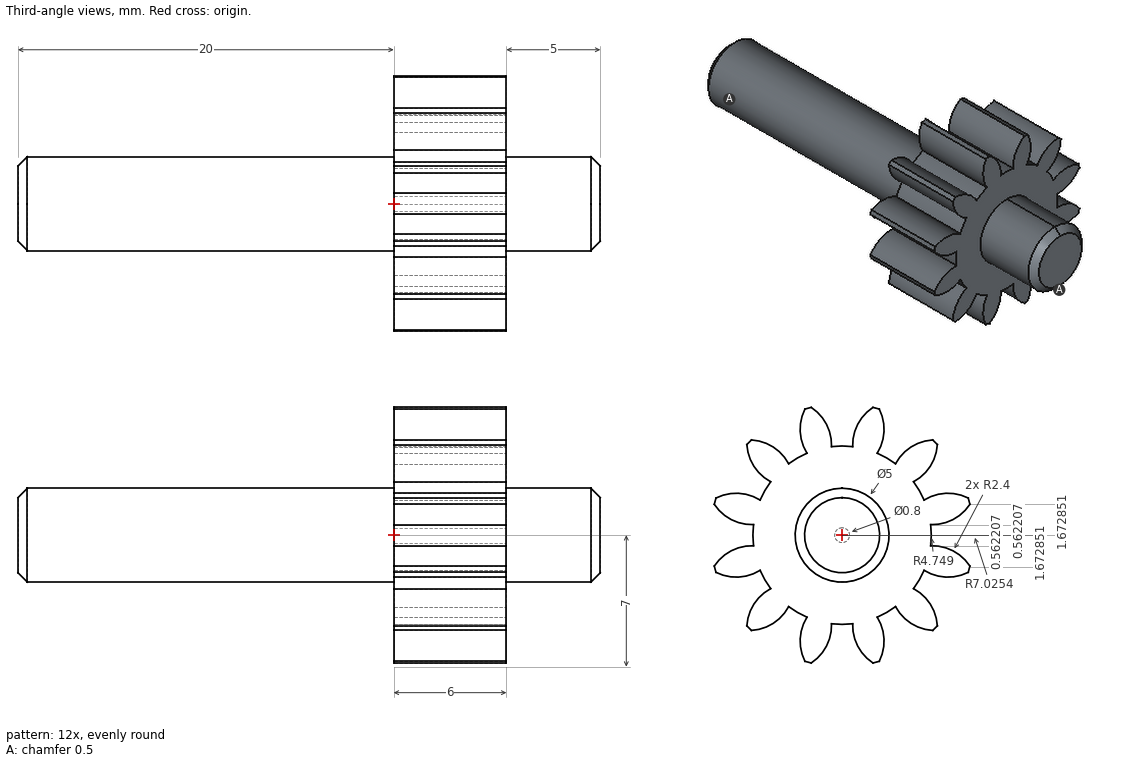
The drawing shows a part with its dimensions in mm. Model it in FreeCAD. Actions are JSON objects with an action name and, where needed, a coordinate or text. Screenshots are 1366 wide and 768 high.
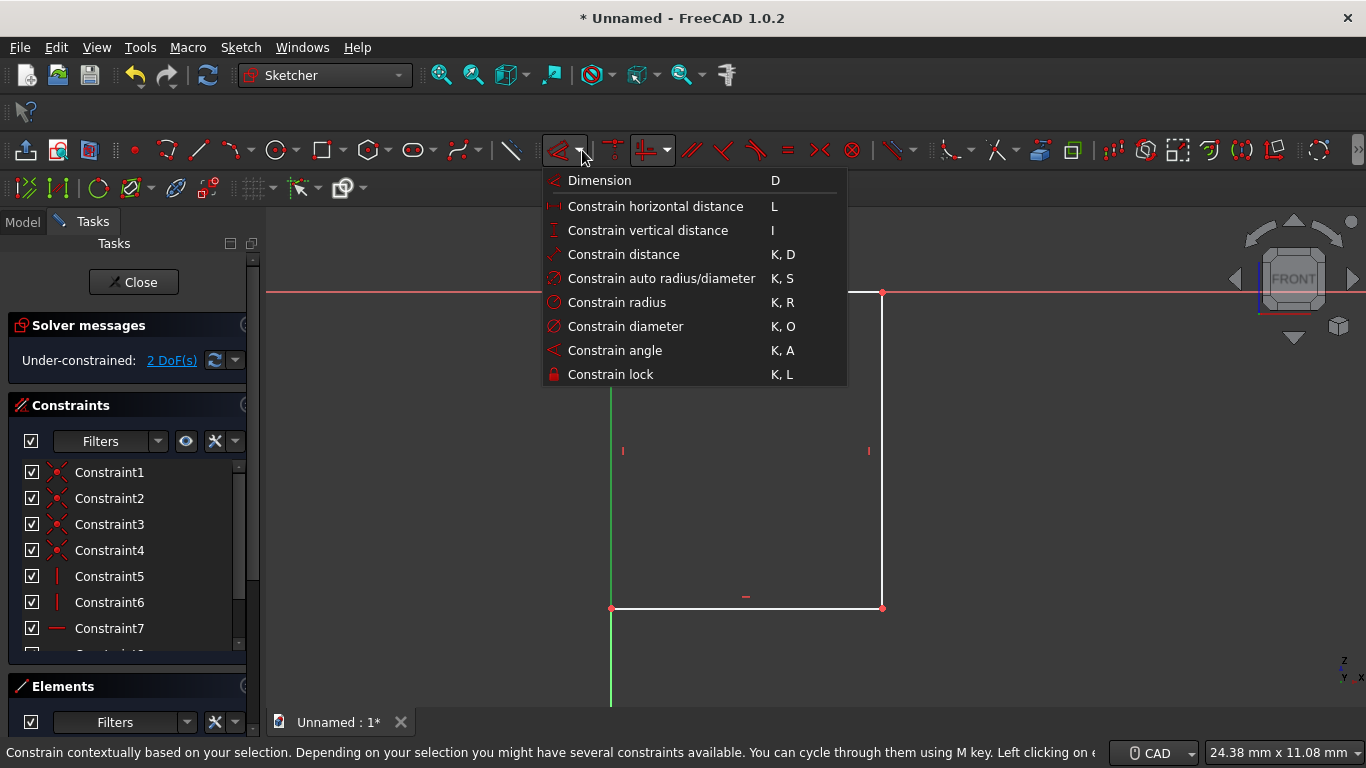
{"action": "left_click", "coordinate": [695, 230]}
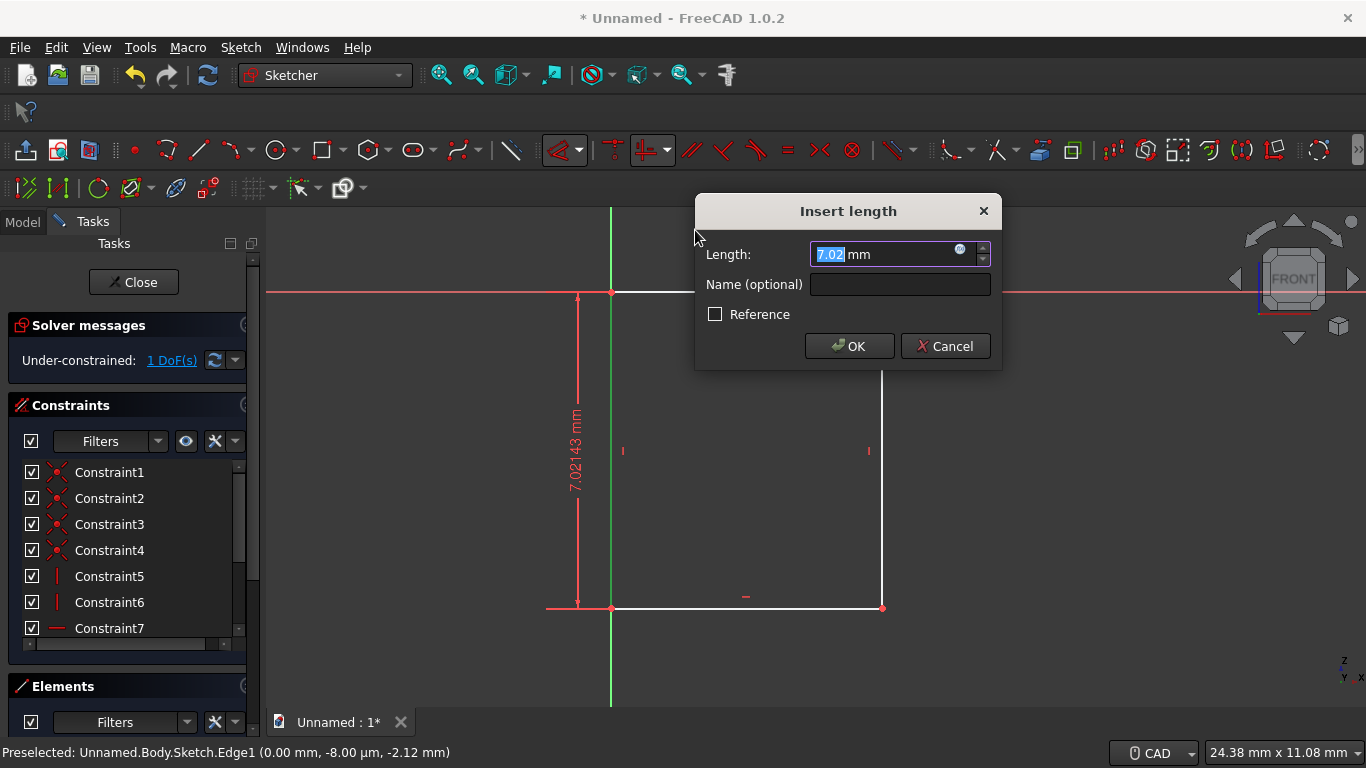
{"action": "type", "text": "7"}
{"action": "key", "text": "Return"}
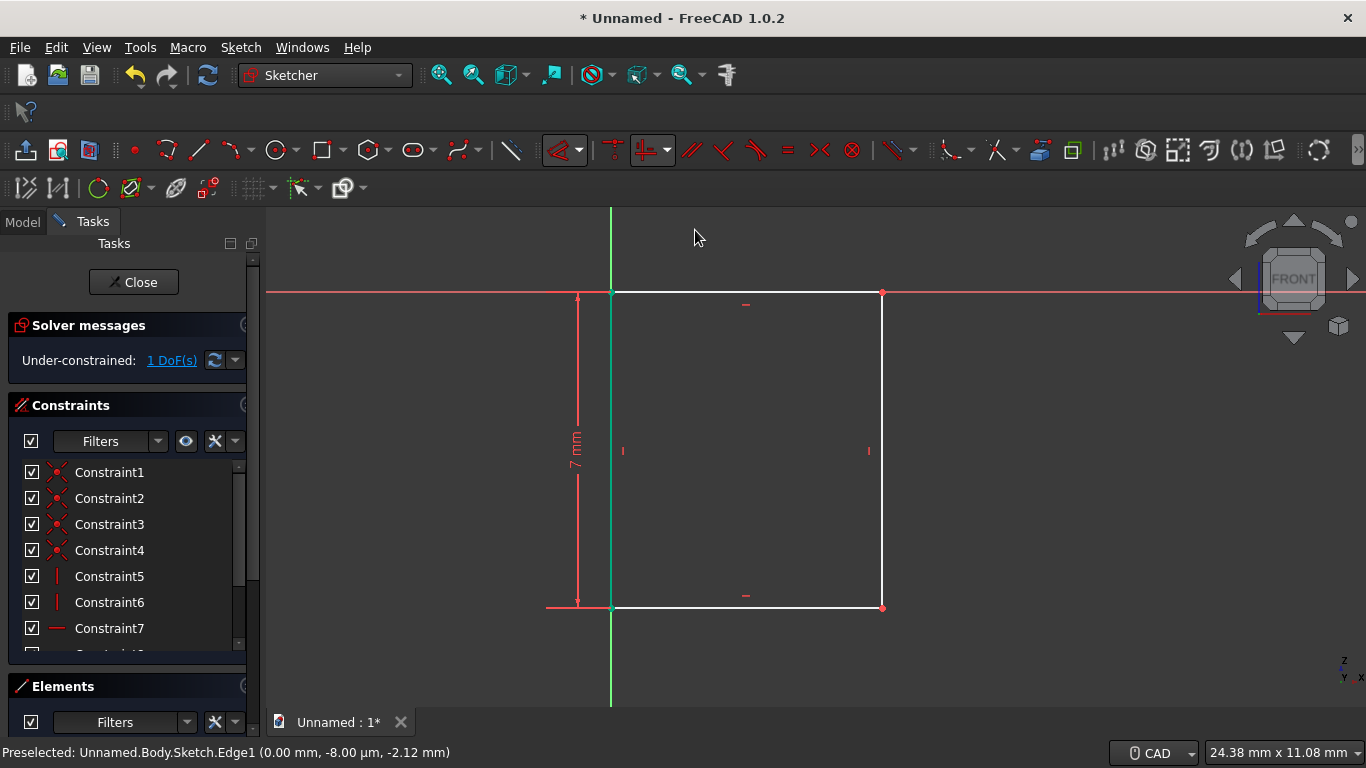
{"action": "left_click", "coordinate": [692, 608]}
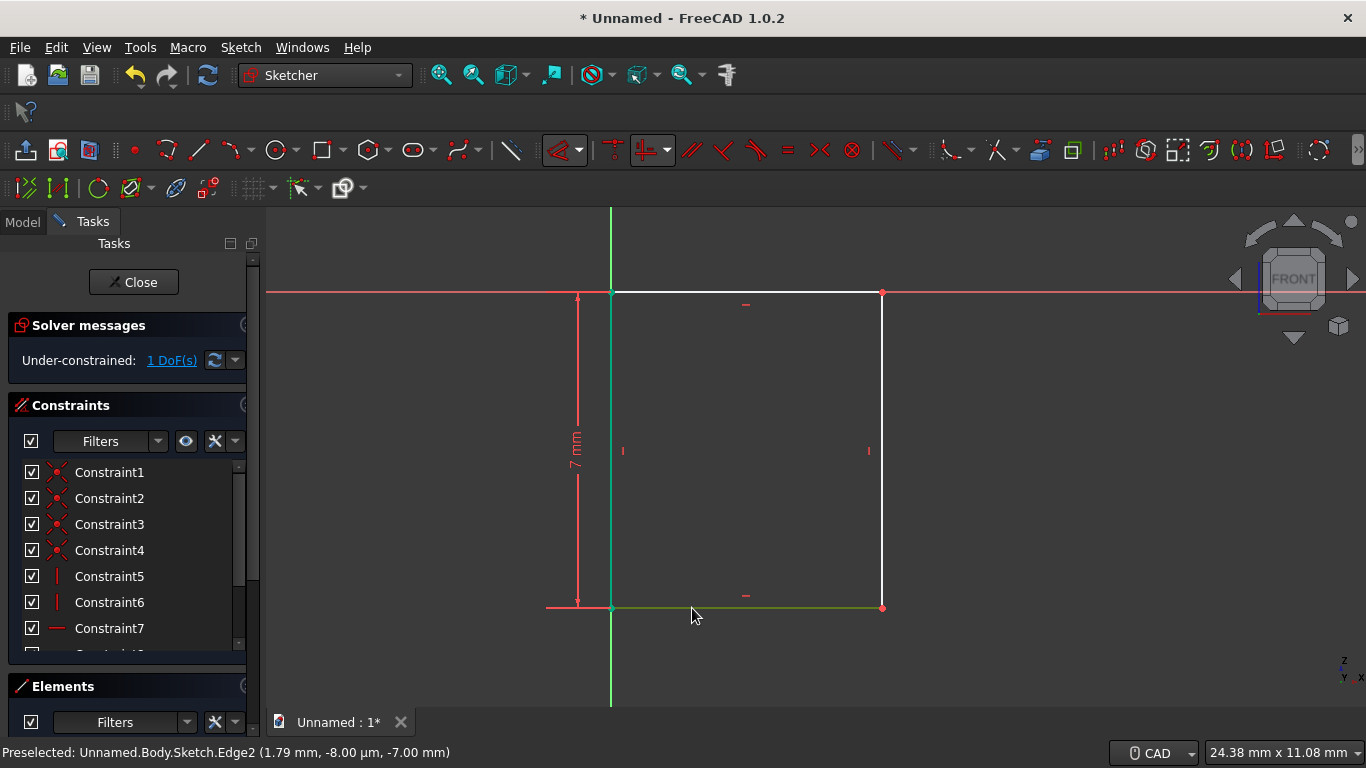
{"action": "key", "text": "l"}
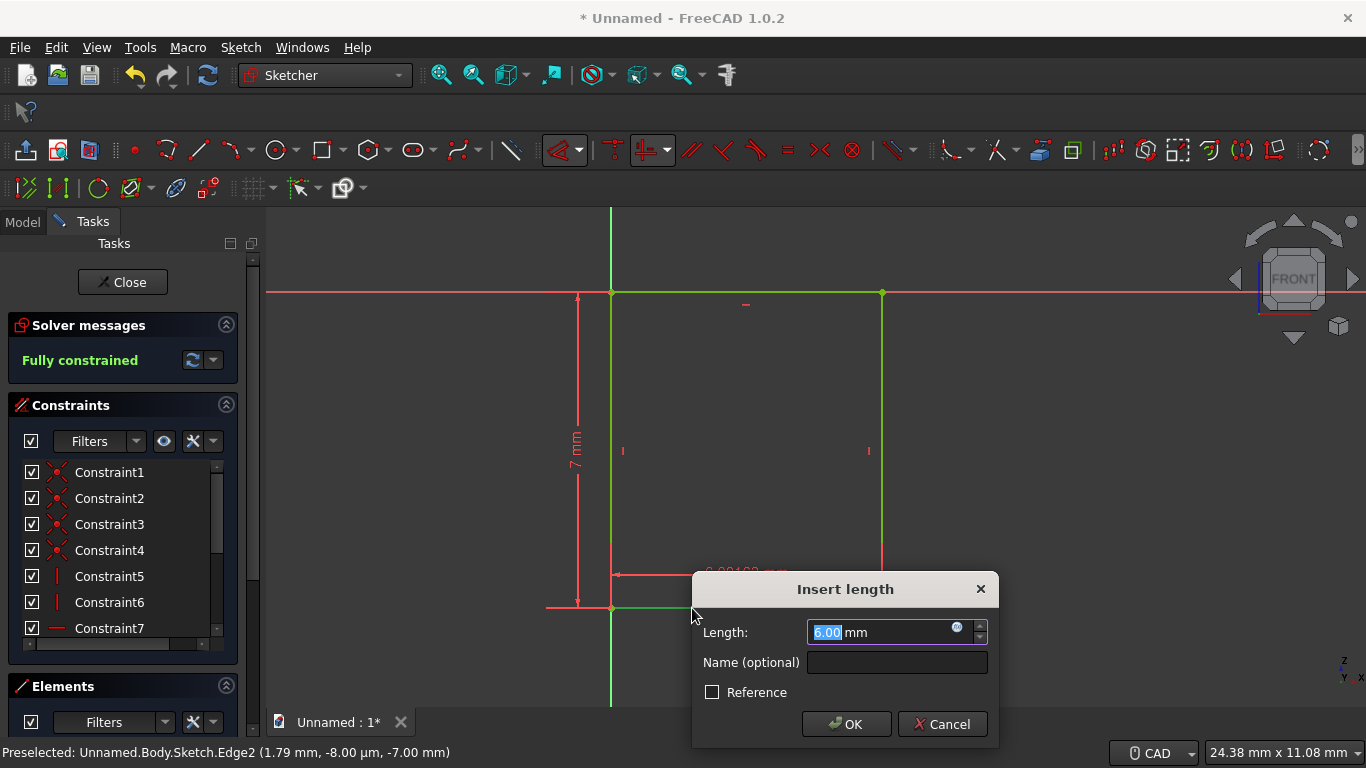
{"action": "type", "text": "6"}
{"action": "key", "text": "Return"}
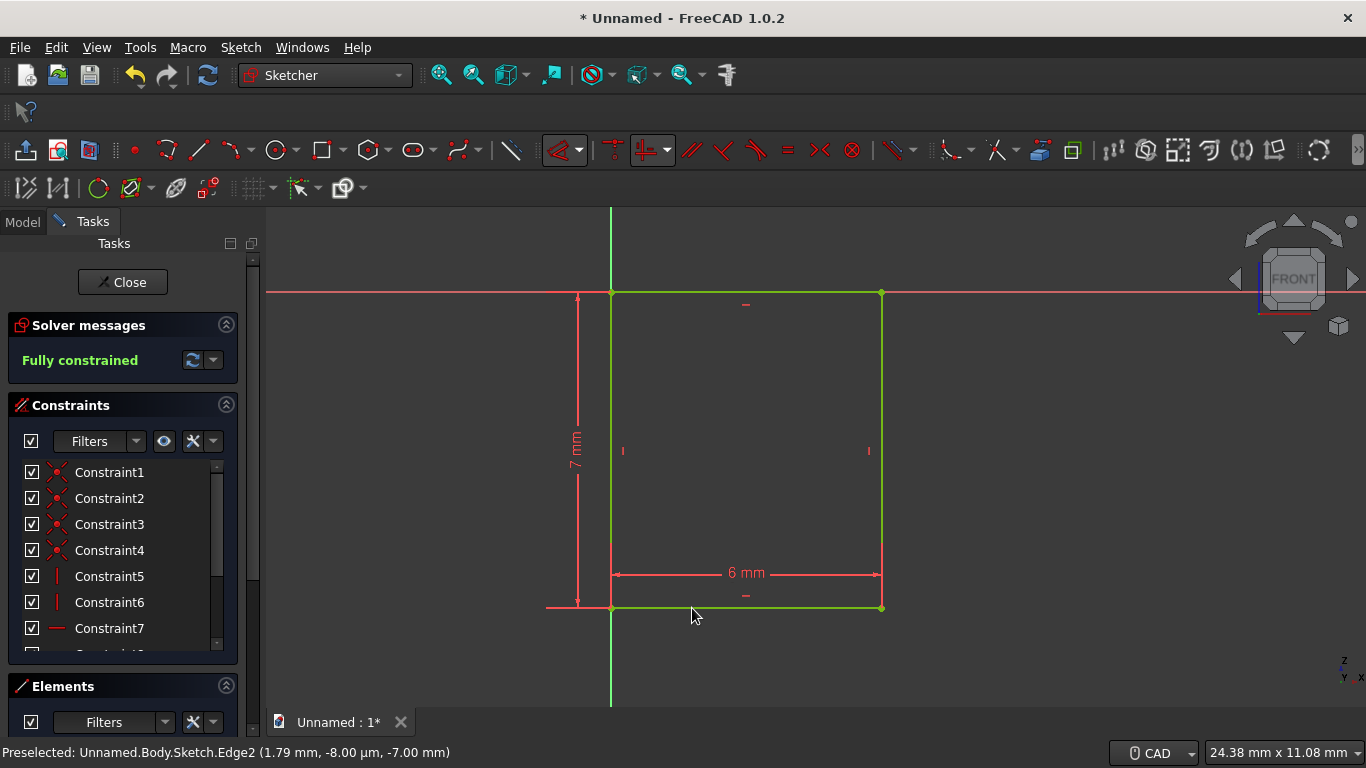
{"action": "left_click", "coordinate": [123, 282]}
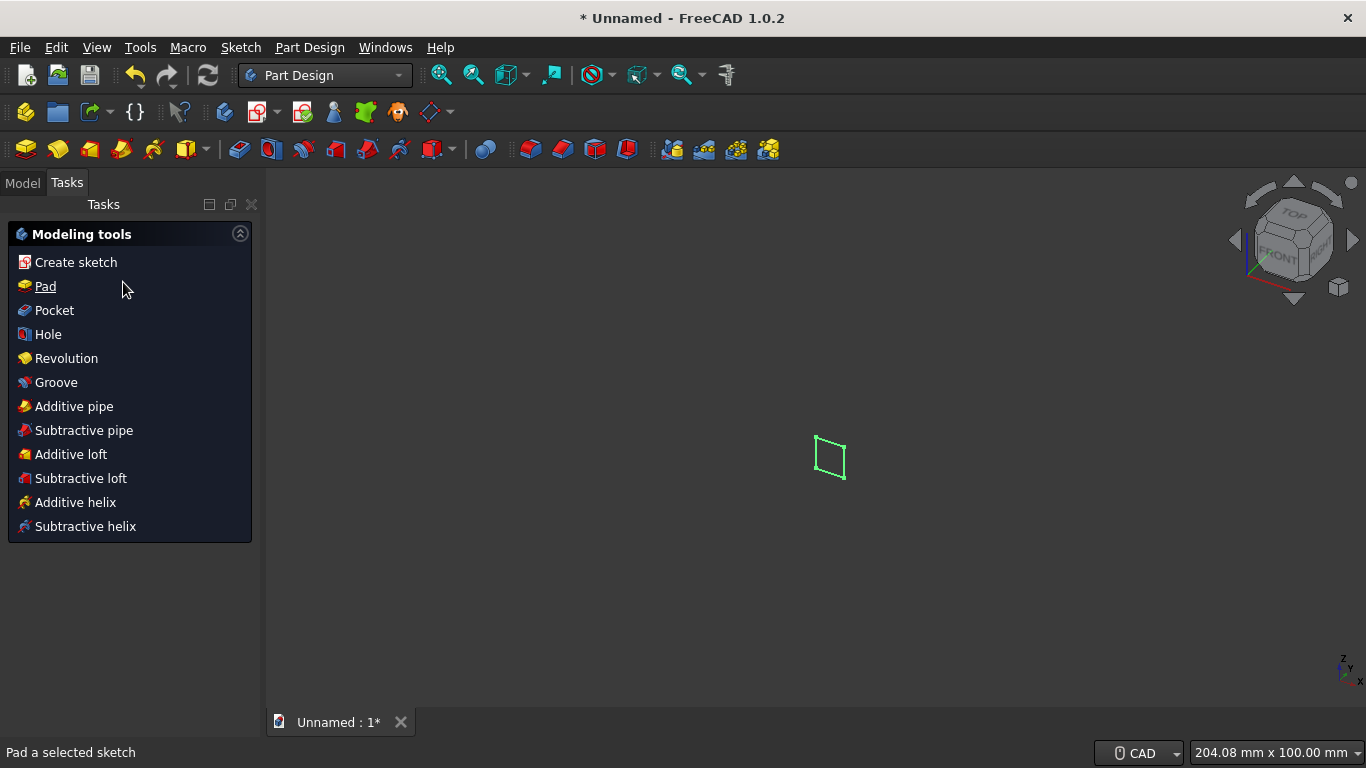
{"action": "left_click", "coordinate": [58, 150]}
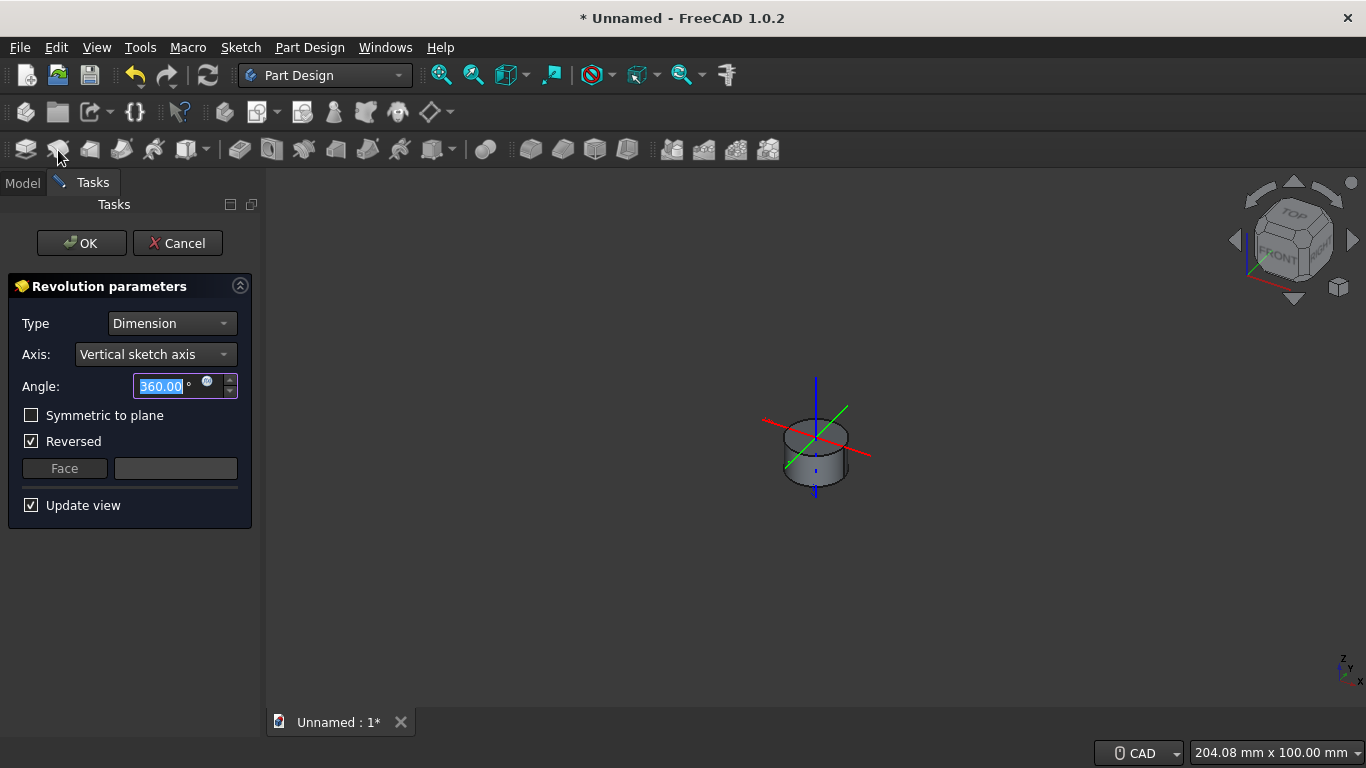
{"action": "left_click", "coordinate": [156, 354]}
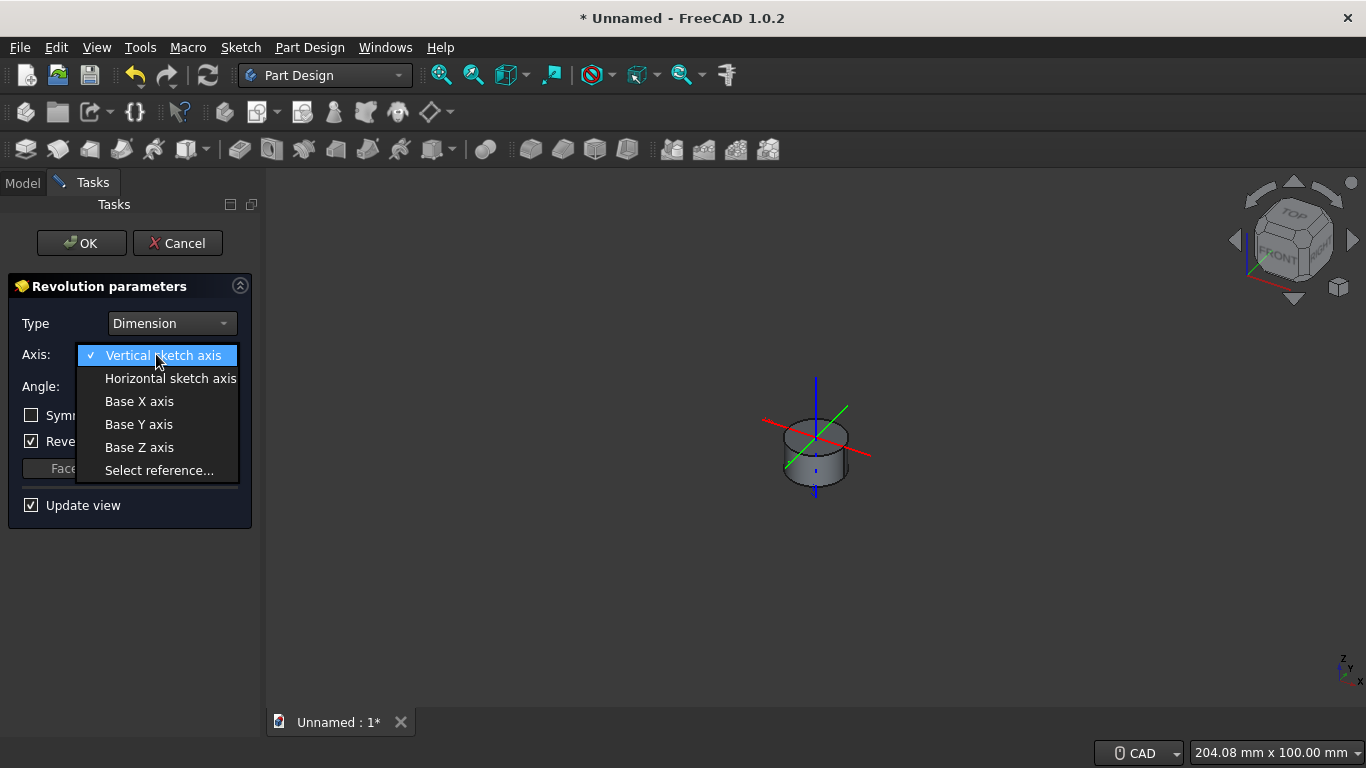
{"action": "left_click", "coordinate": [156, 378]}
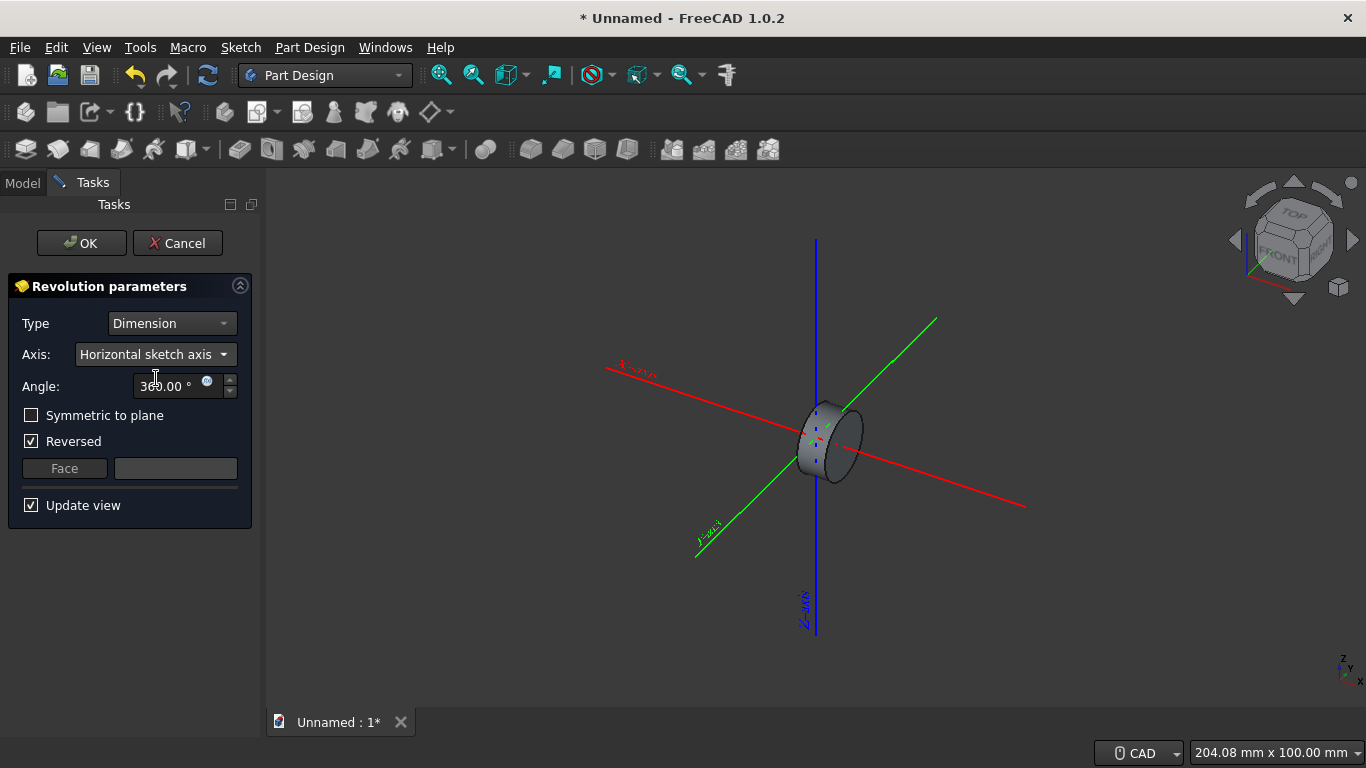
{"action": "left_click", "coordinate": [82, 243]}